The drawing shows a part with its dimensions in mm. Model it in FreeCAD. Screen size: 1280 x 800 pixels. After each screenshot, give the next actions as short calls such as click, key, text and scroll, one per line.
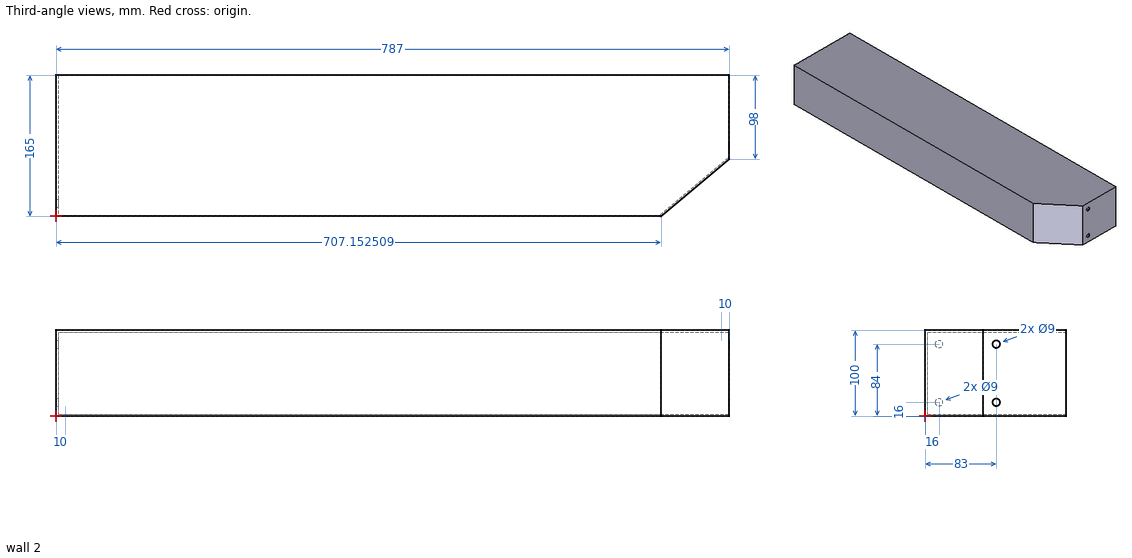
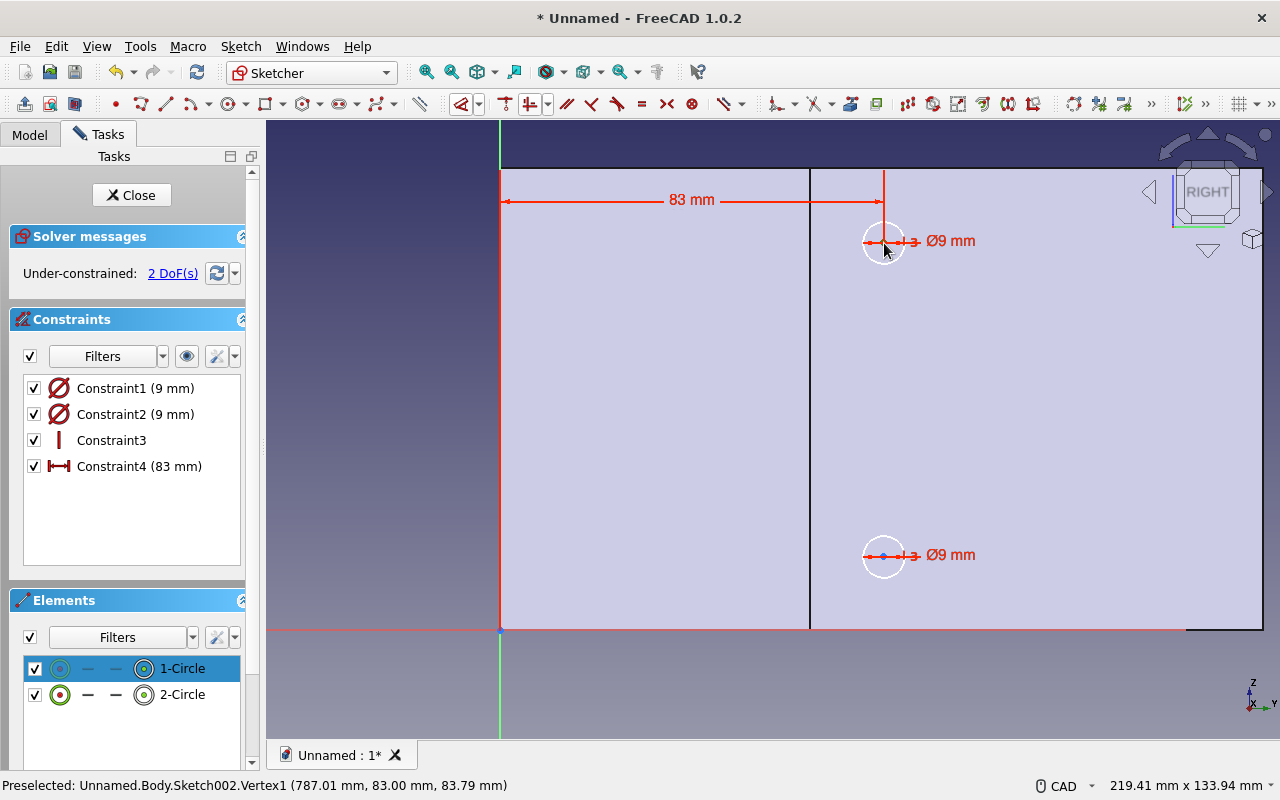
click(478, 104)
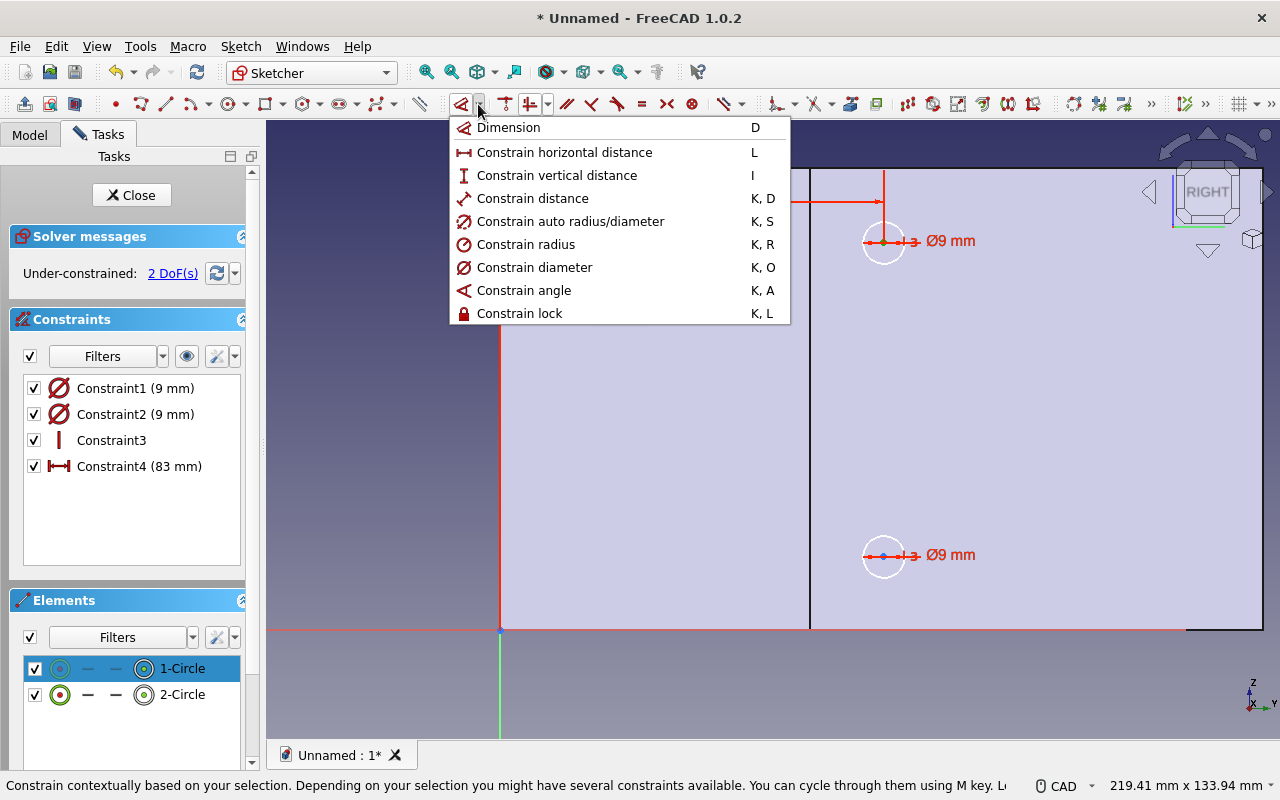
click(620, 176)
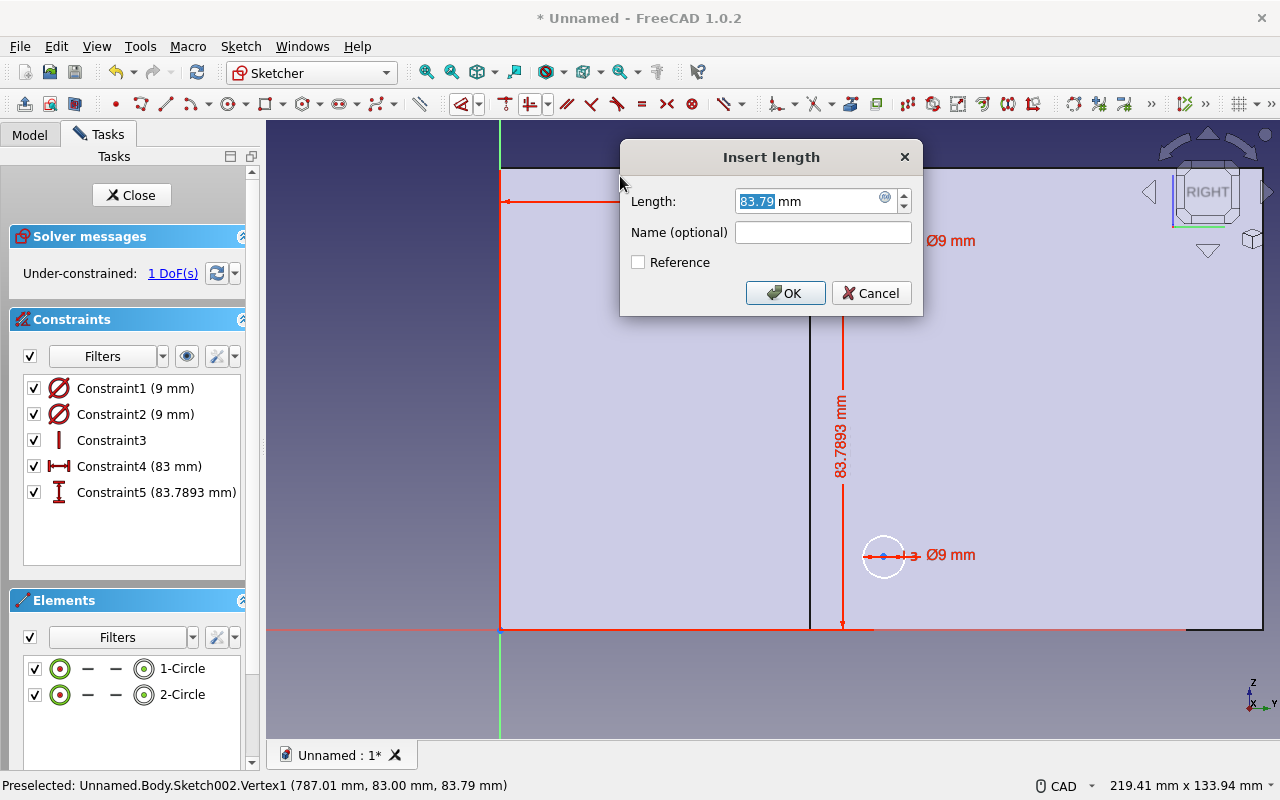
text(84)
key(Return)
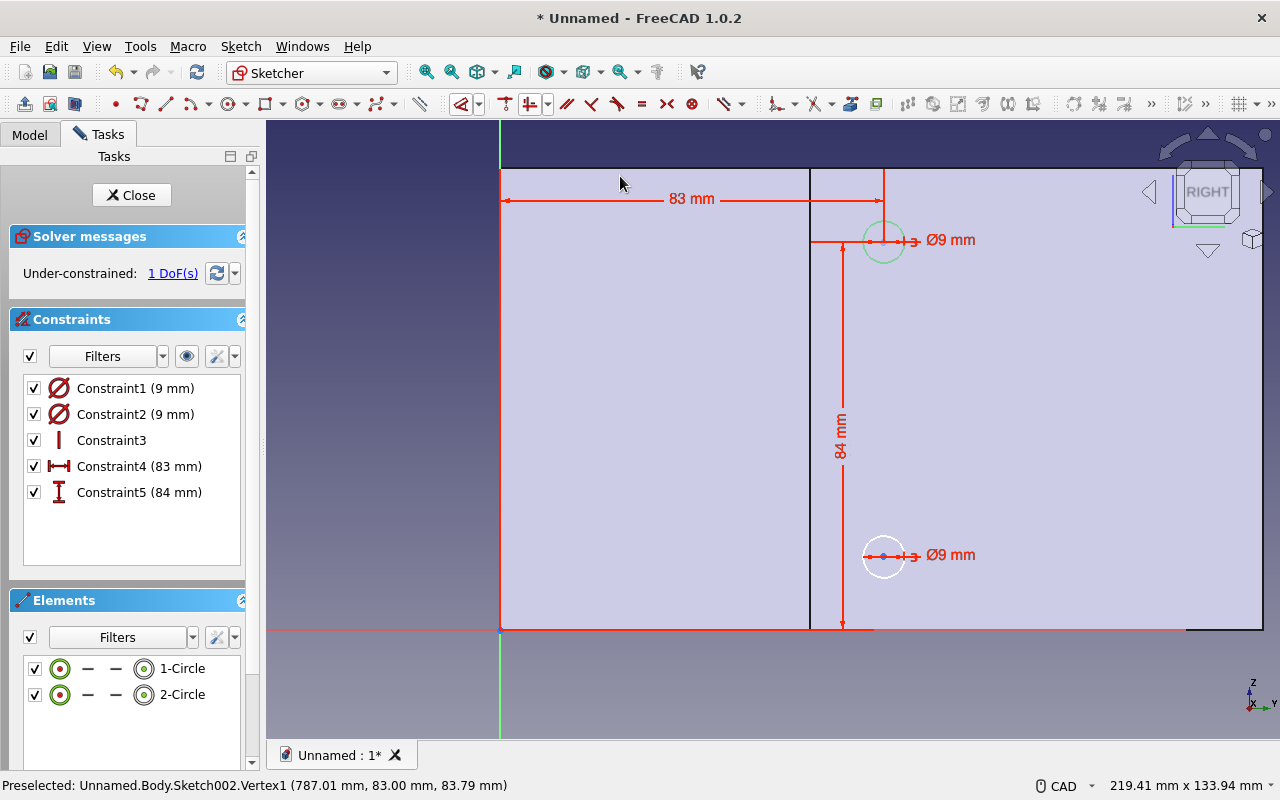
click(884, 557)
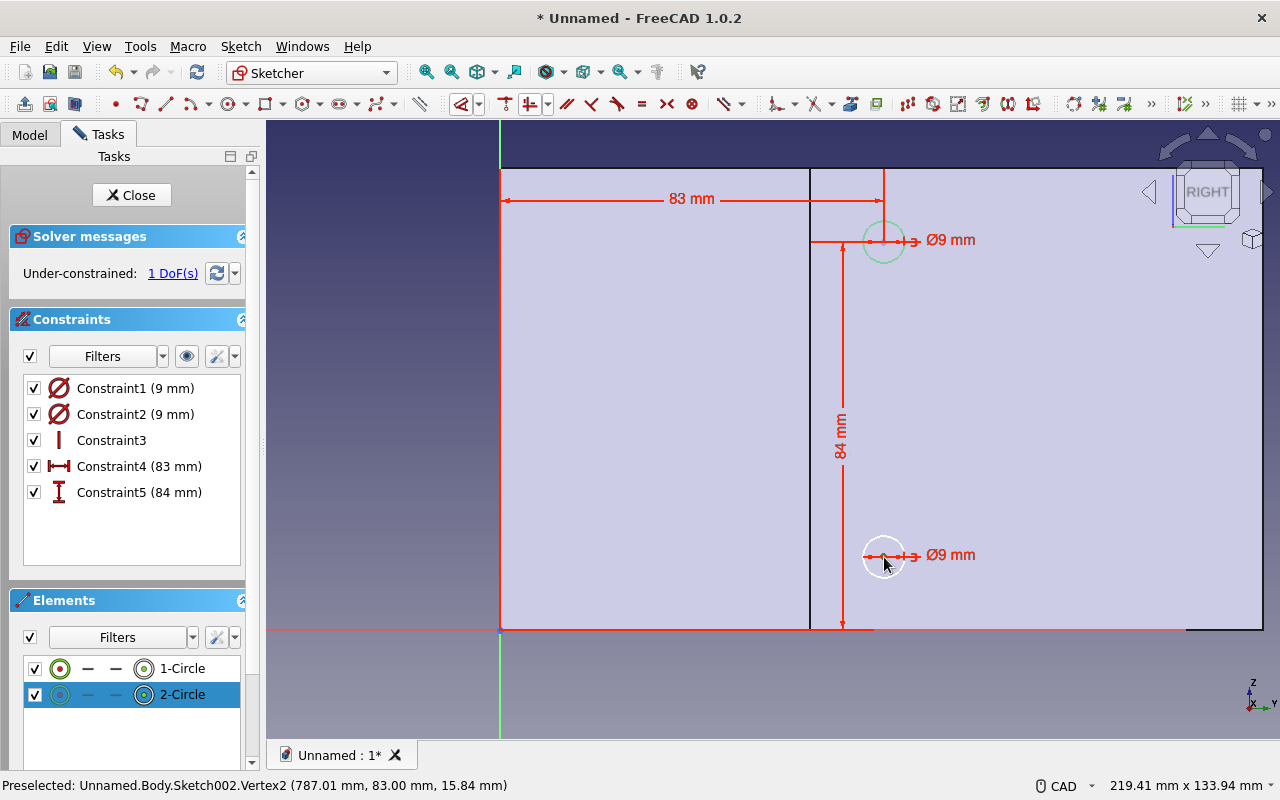
click(478, 104)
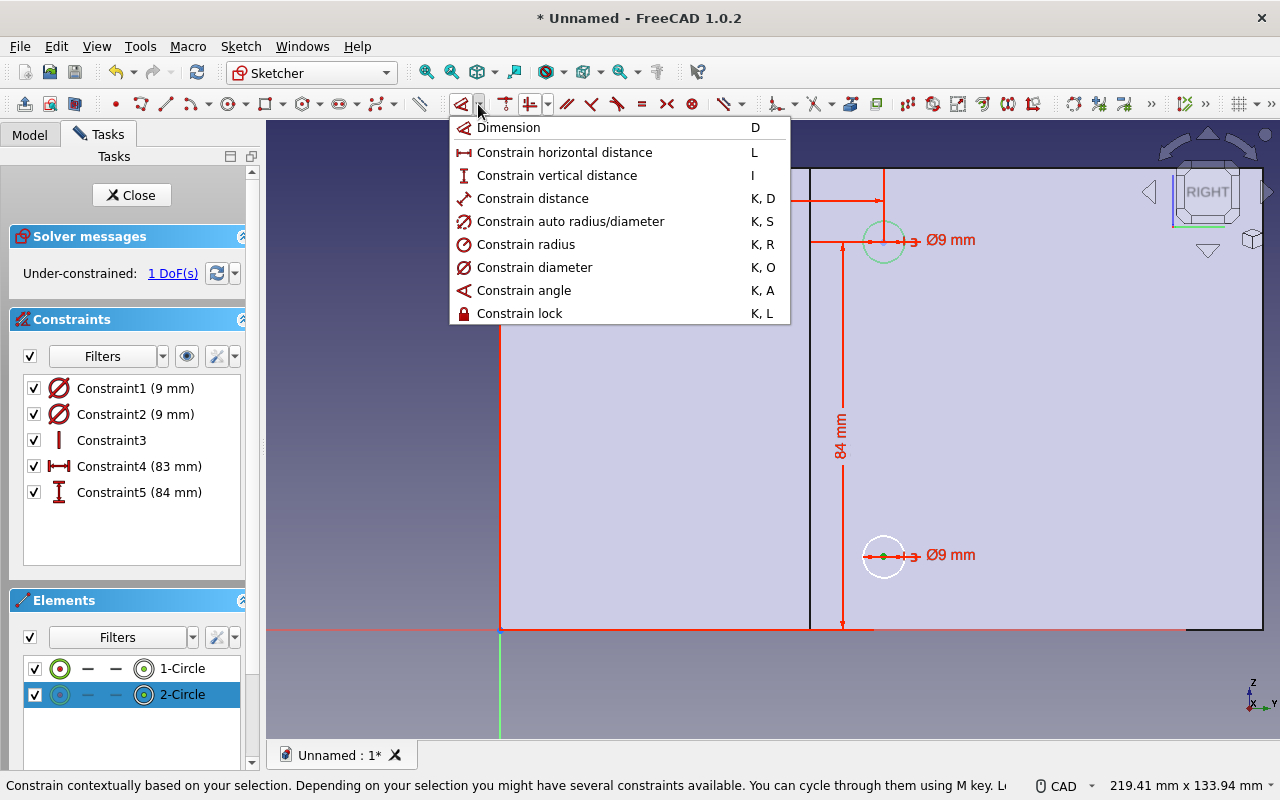
click(620, 176)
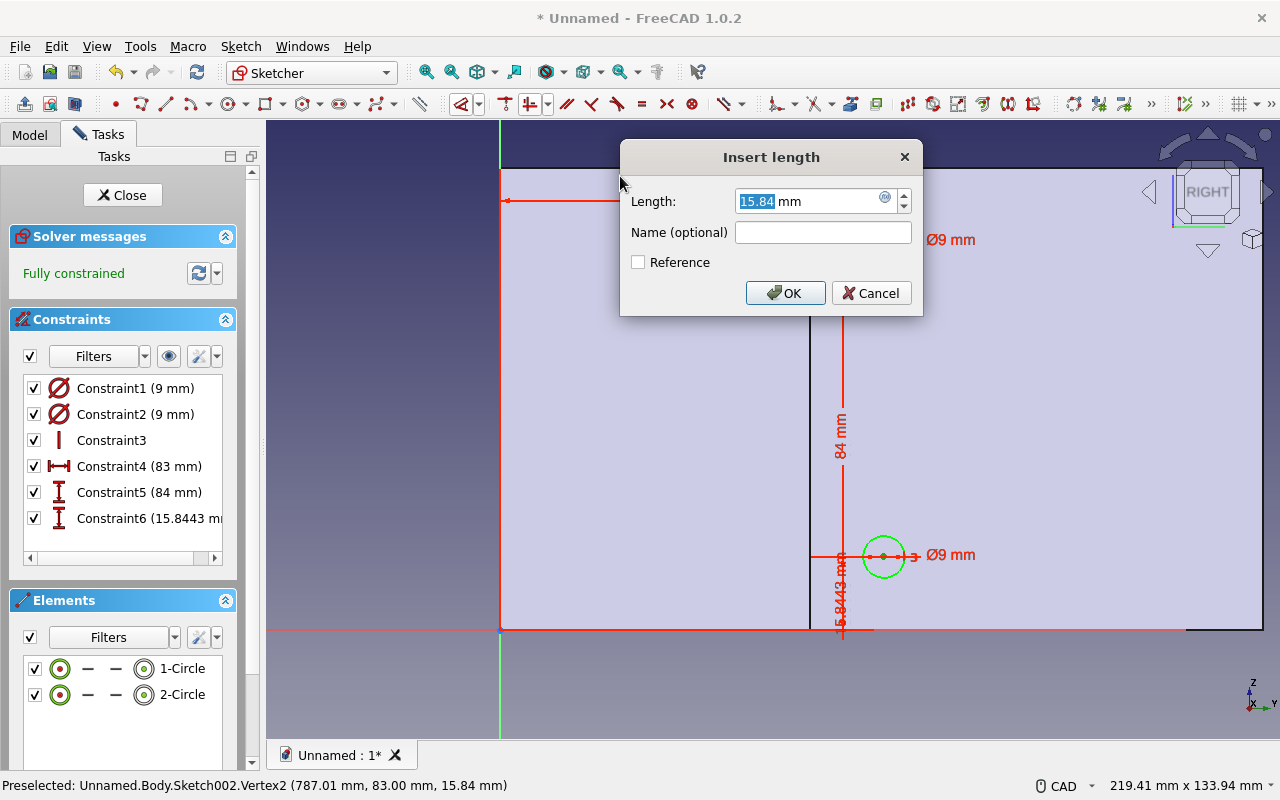
text(16)
key(Return)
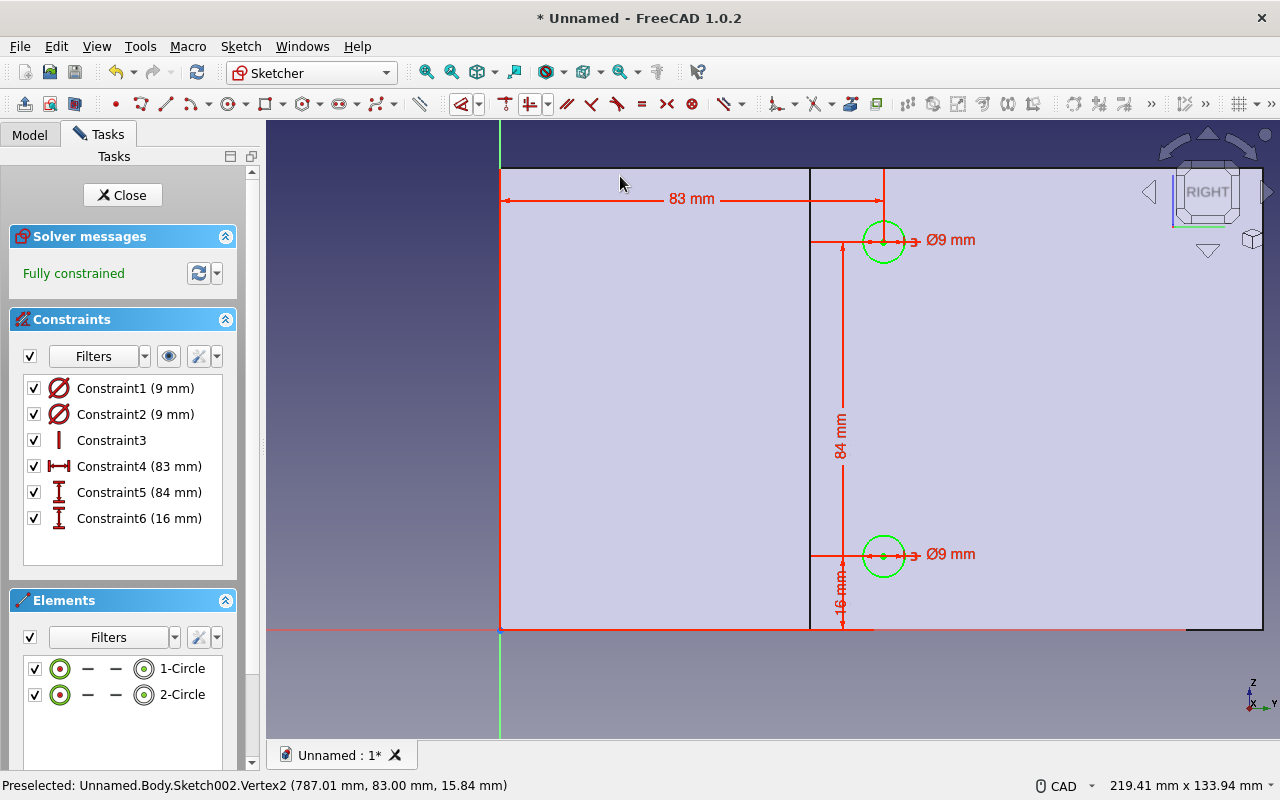
click(123, 195)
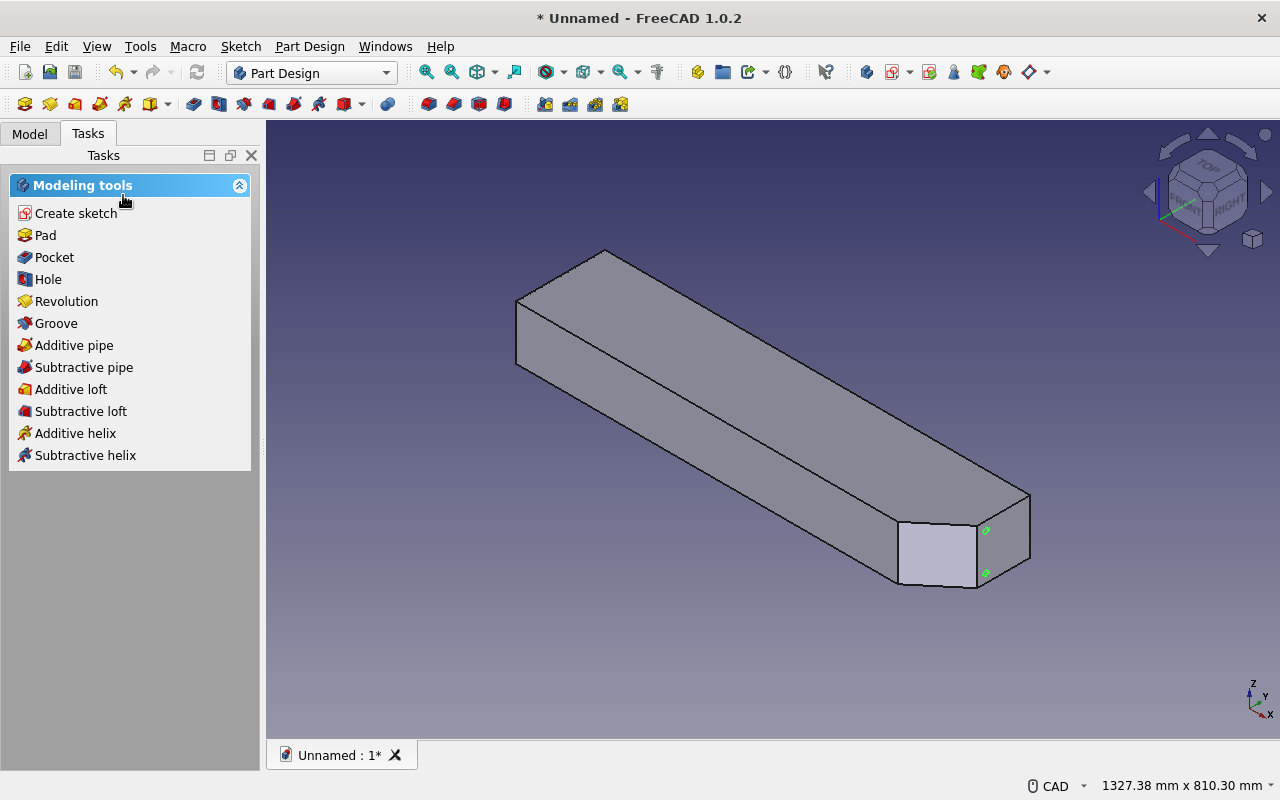
click(194, 104)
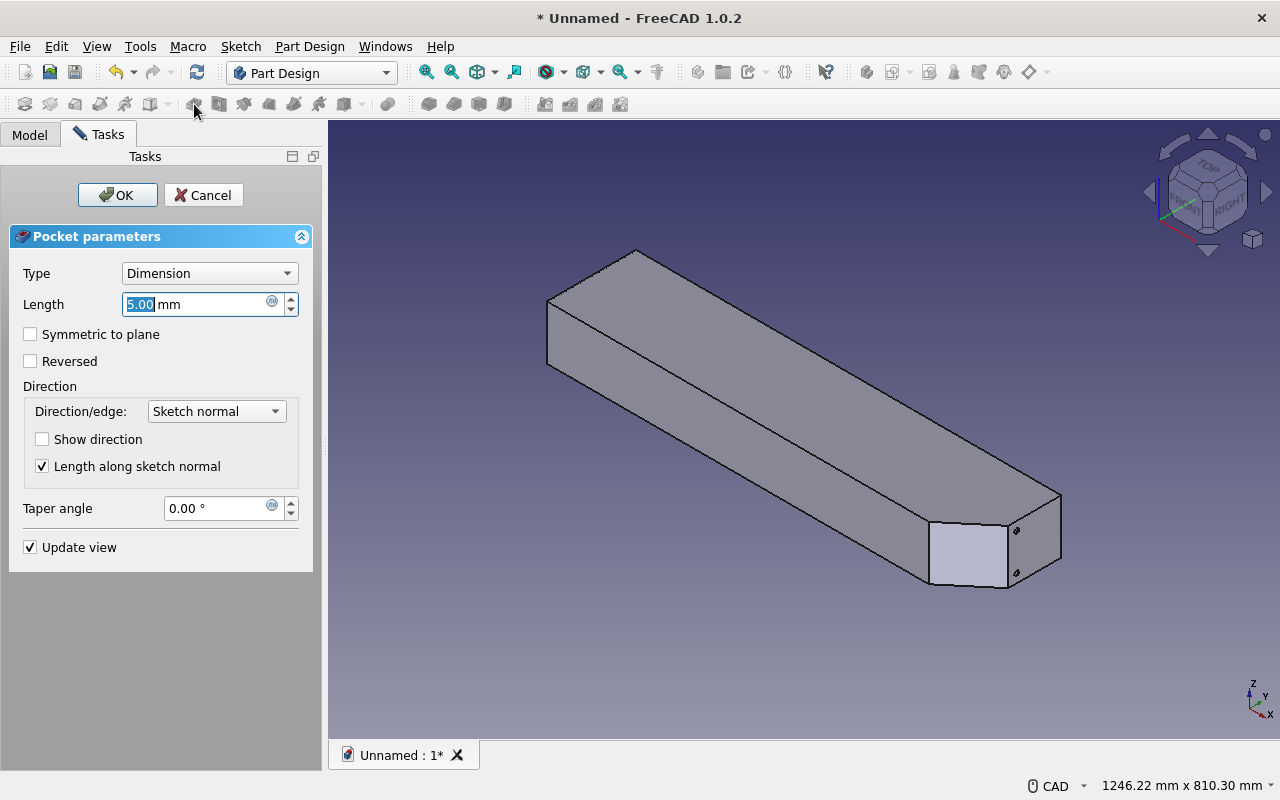
text(10)
key(Tab)